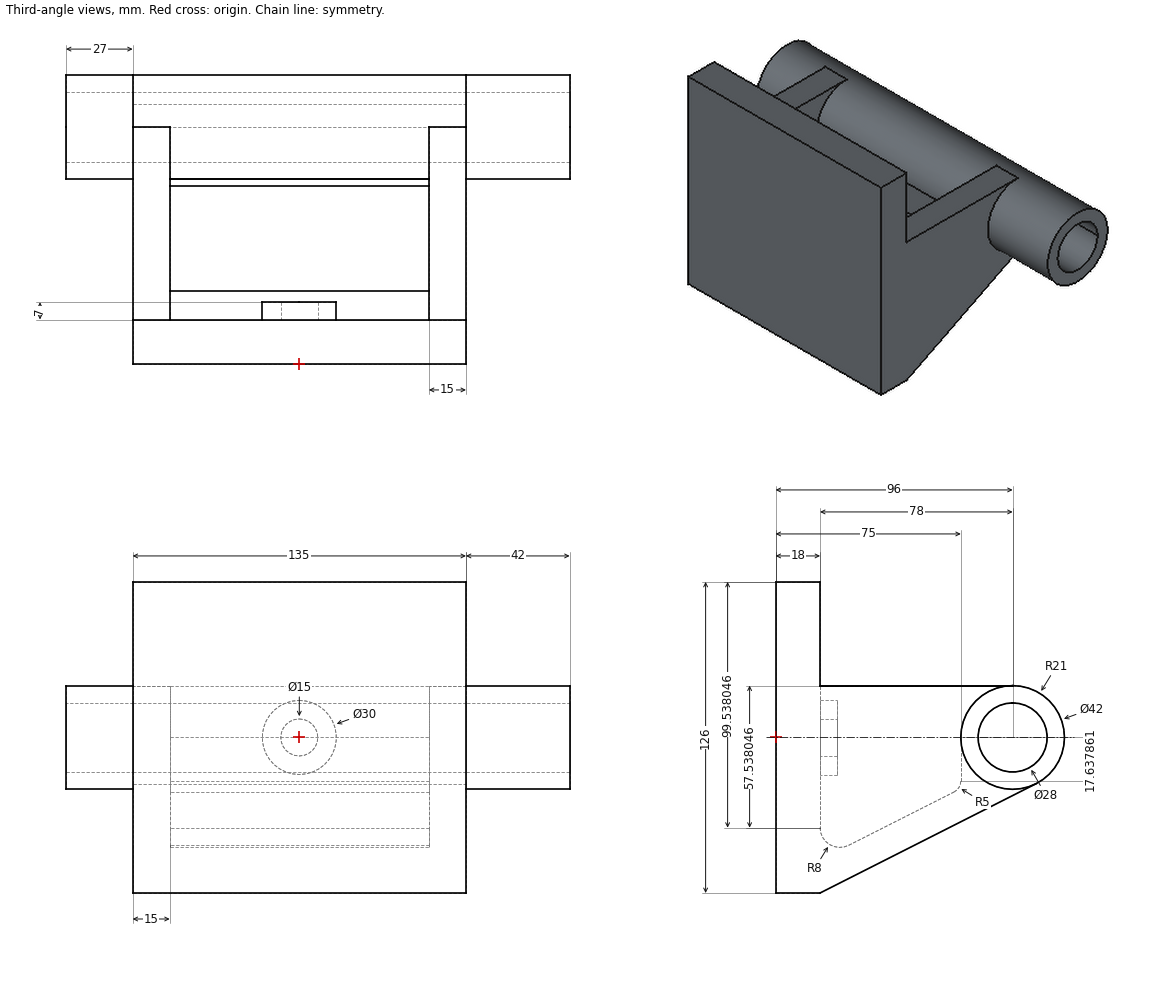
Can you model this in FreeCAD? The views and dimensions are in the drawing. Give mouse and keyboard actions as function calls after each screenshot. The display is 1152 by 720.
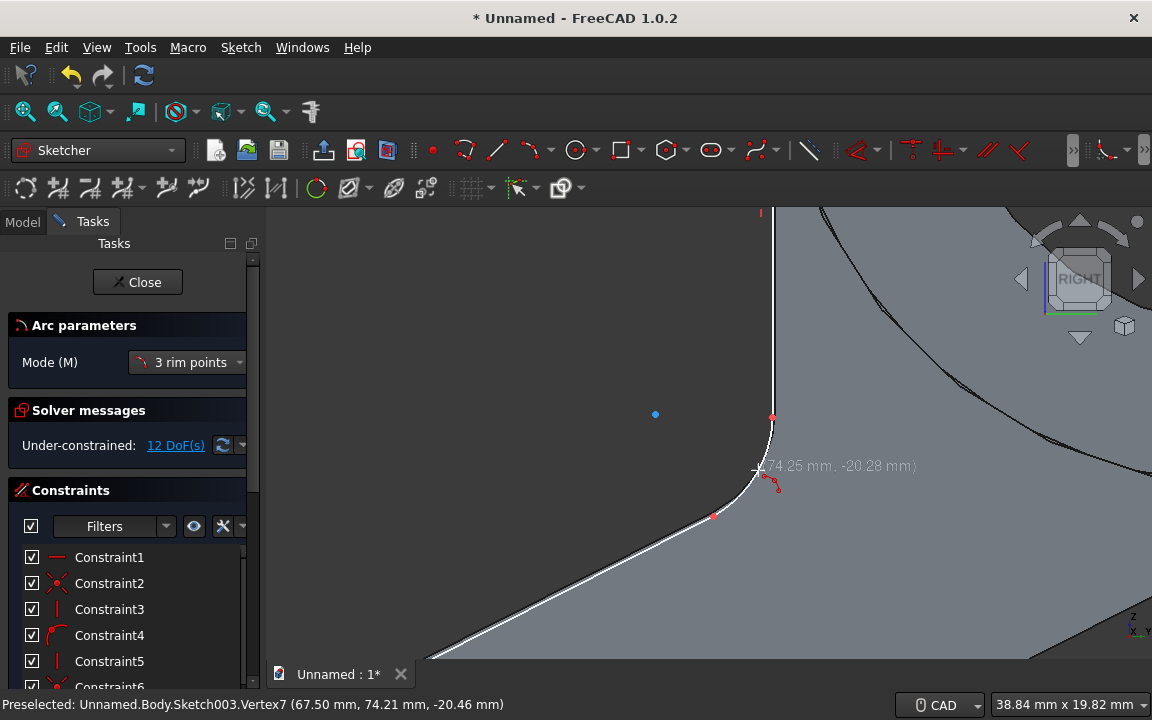
scroll(762, 475, down, 8)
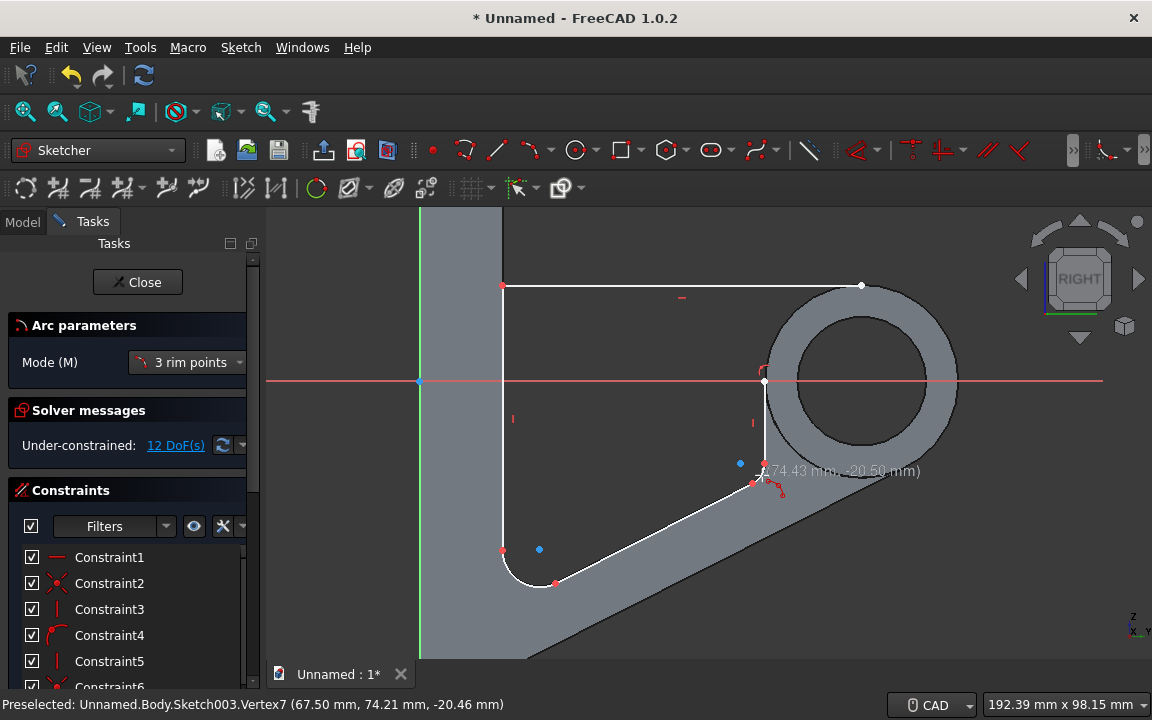
click(765, 381)
click(862, 286)
click(793, 313)
key(Escape)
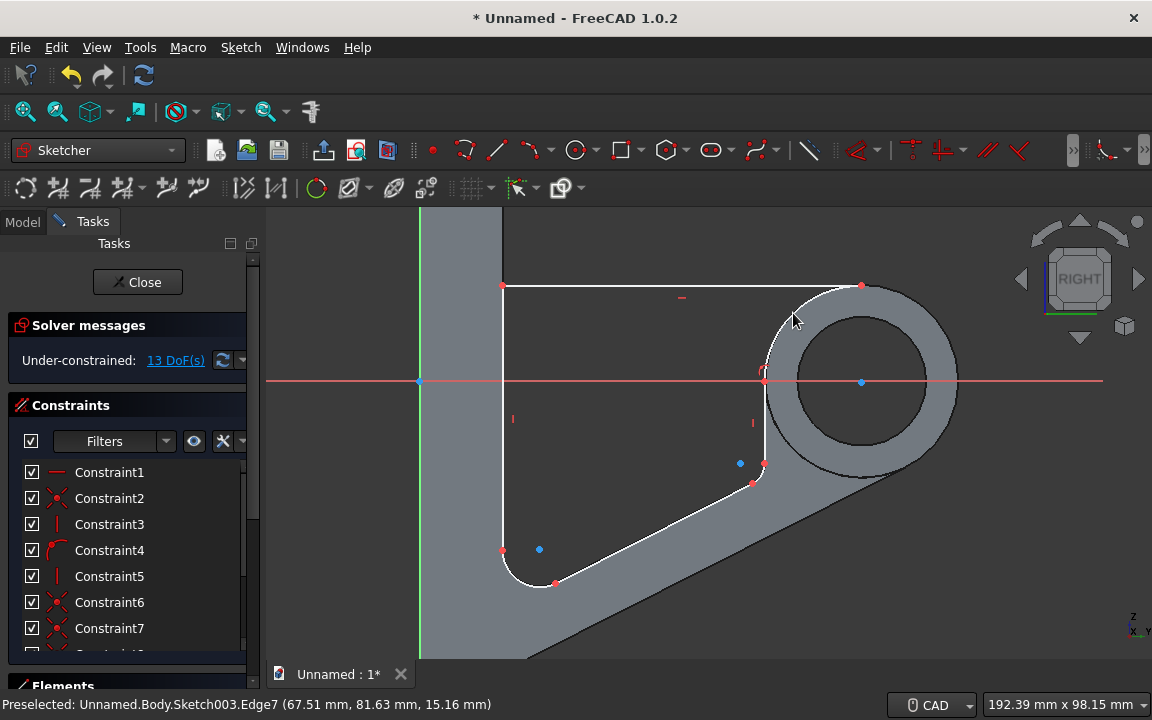
click(754, 286)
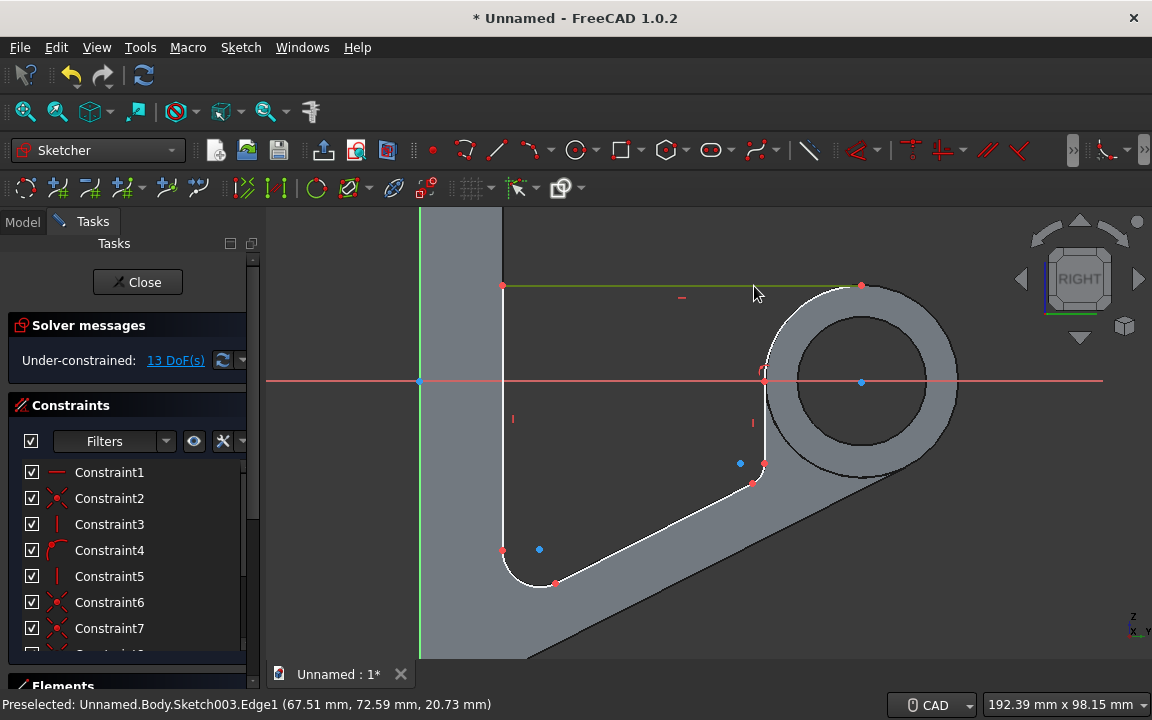
scroll(818, 296, up, 2)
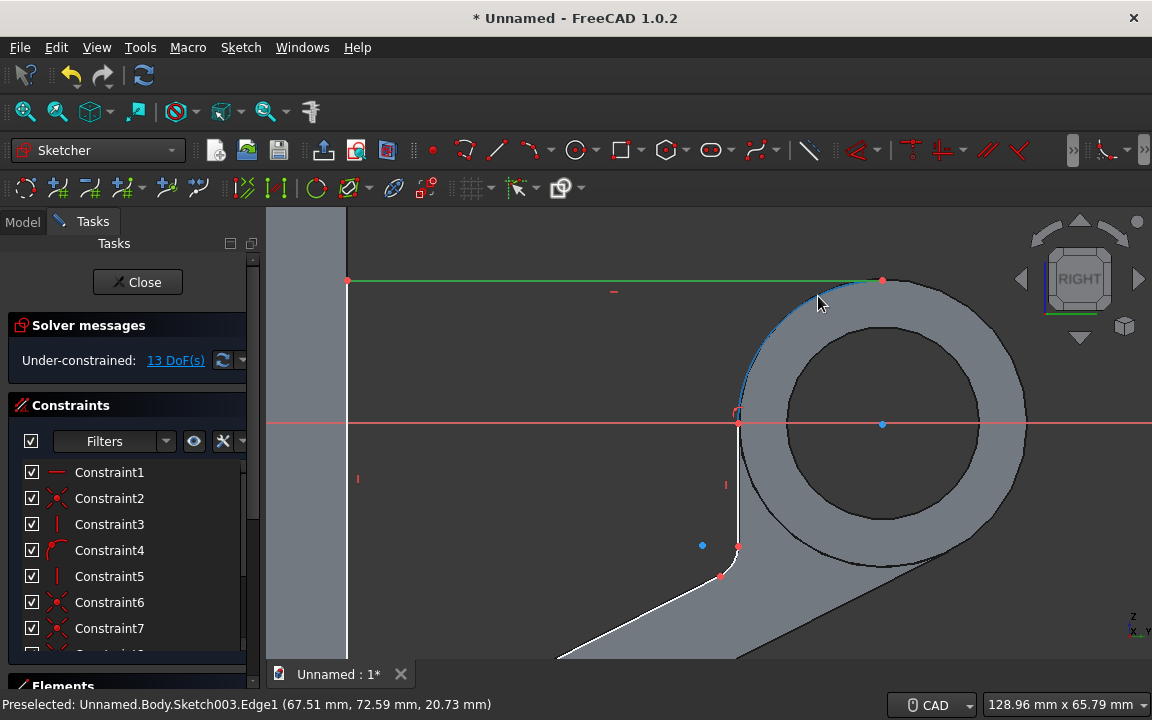
click(818, 296)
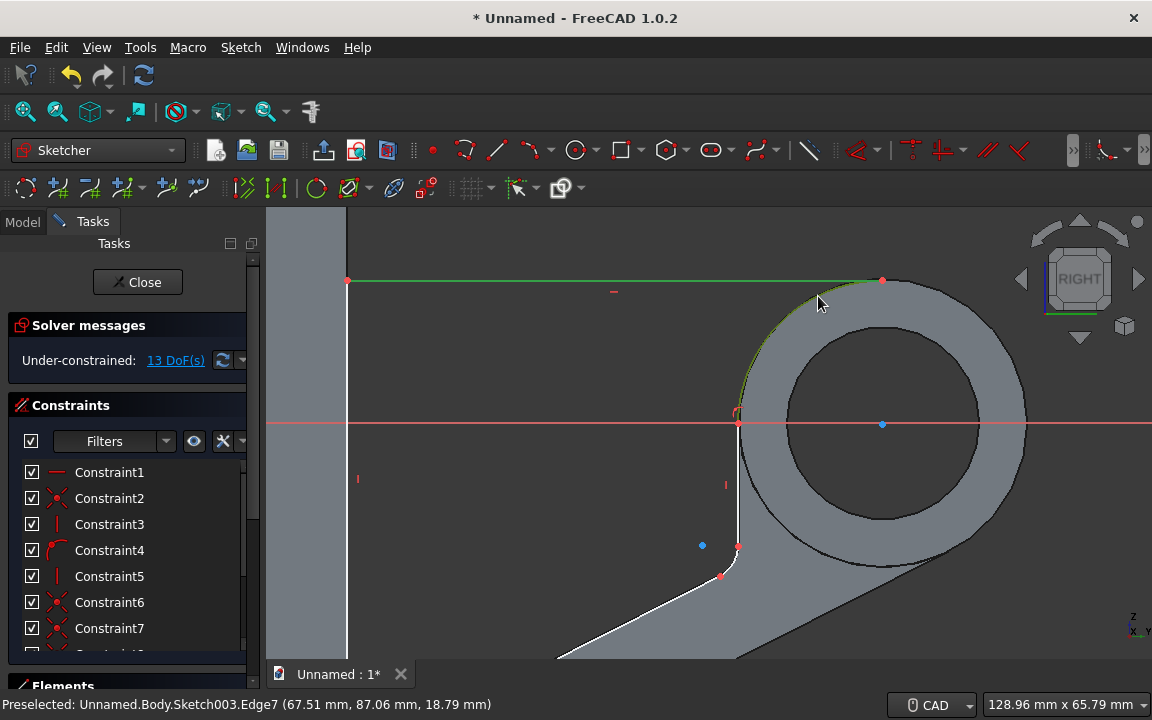
key(t)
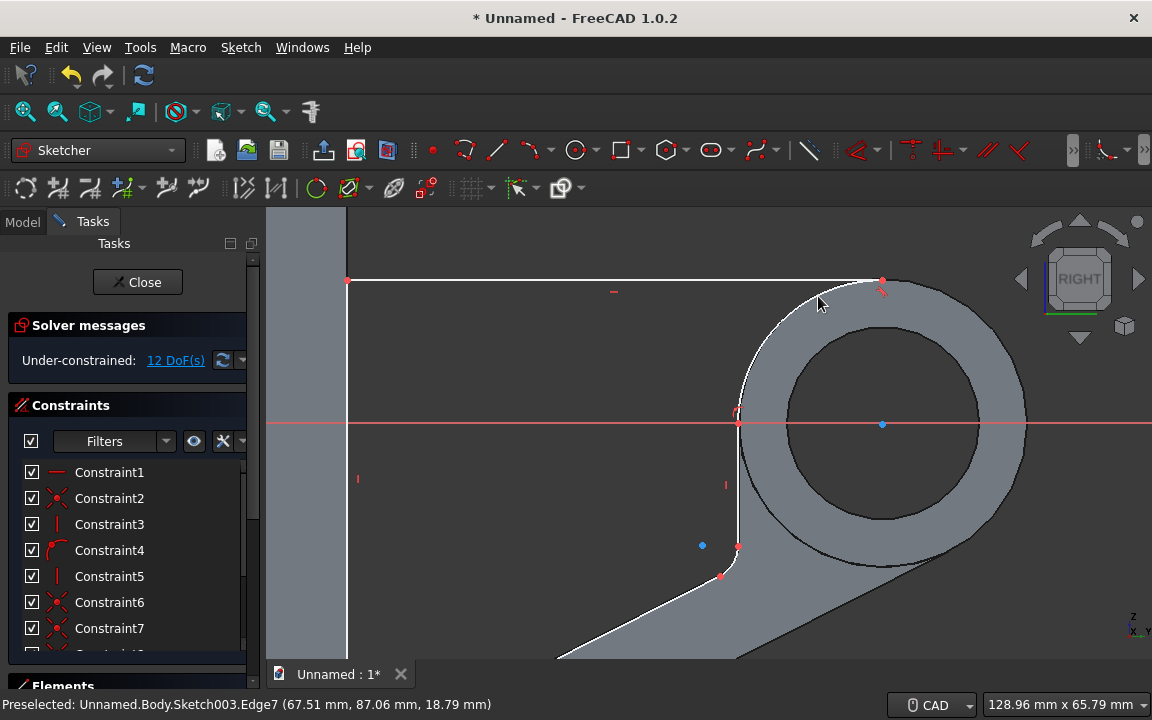
click(347, 399)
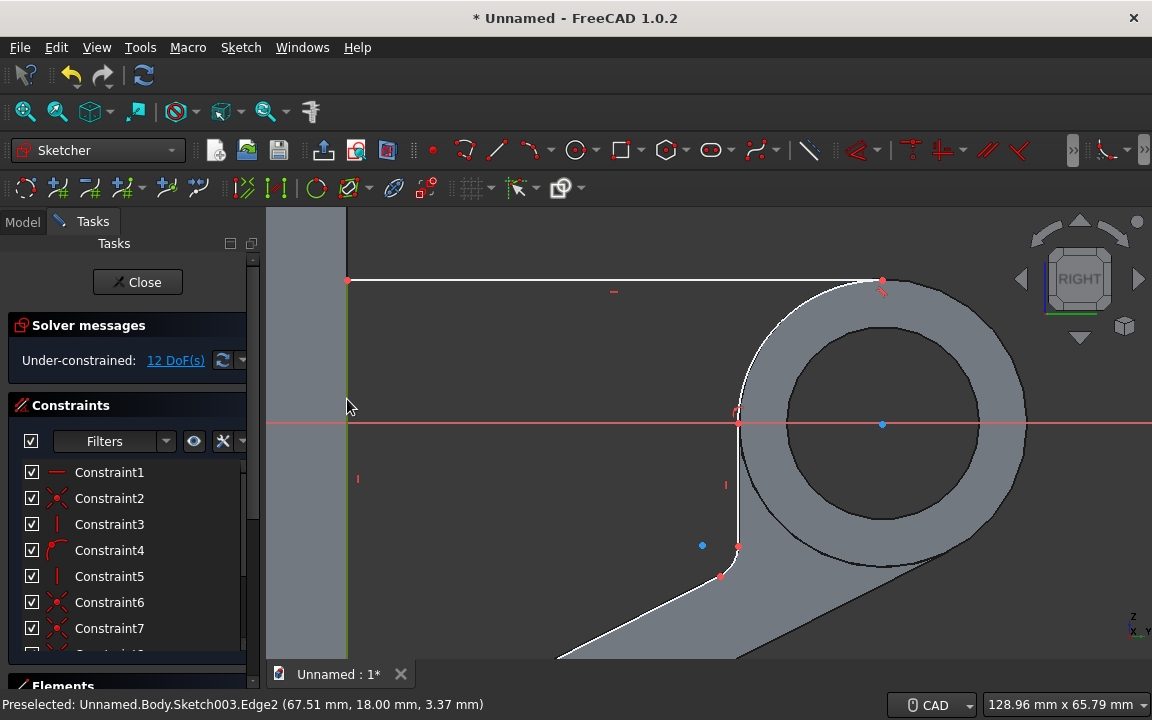
scroll(818, 295, down, 2)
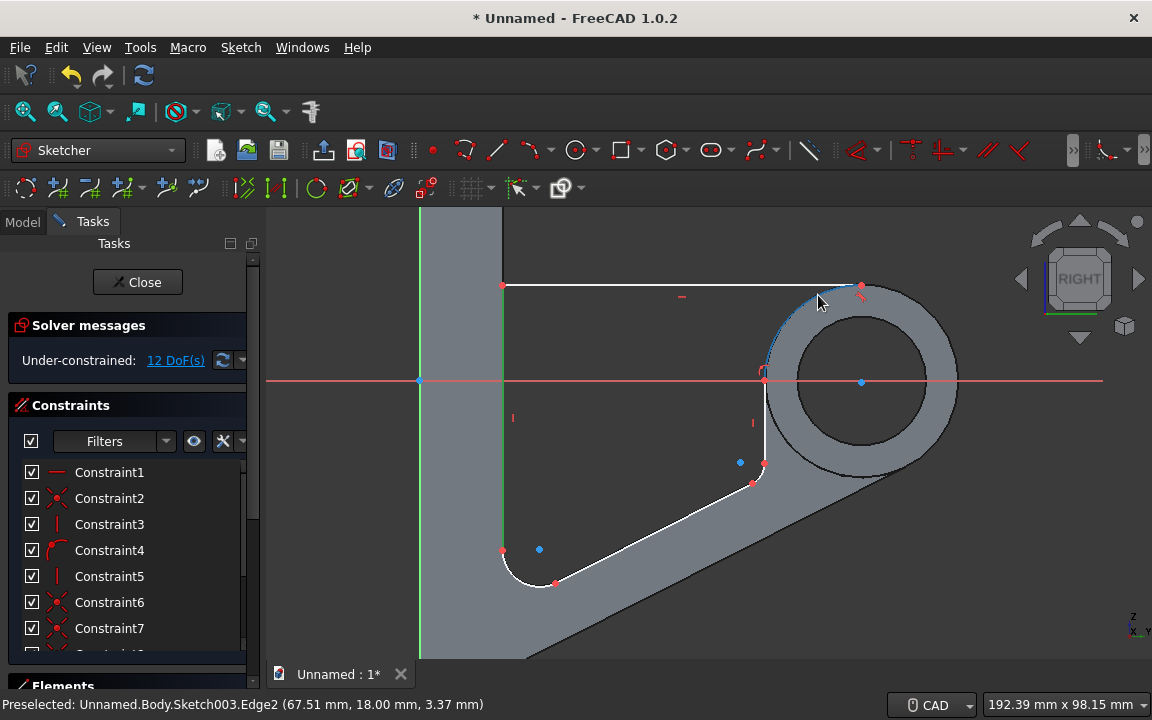
click(510, 571)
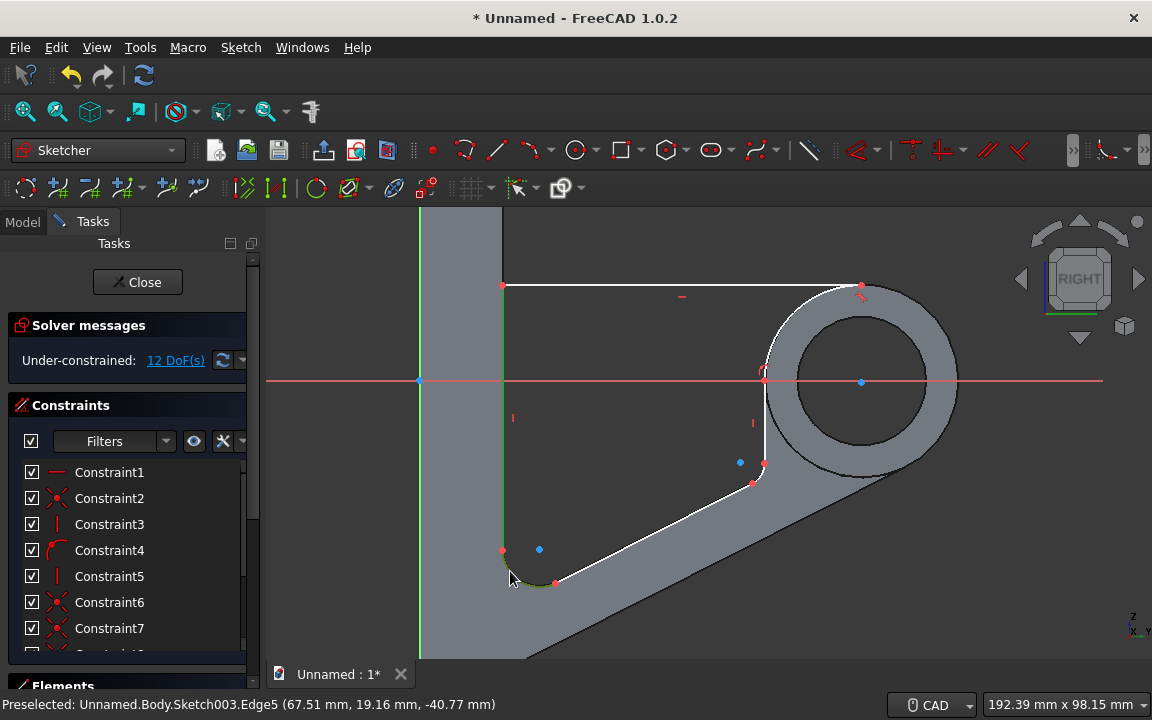
key(t)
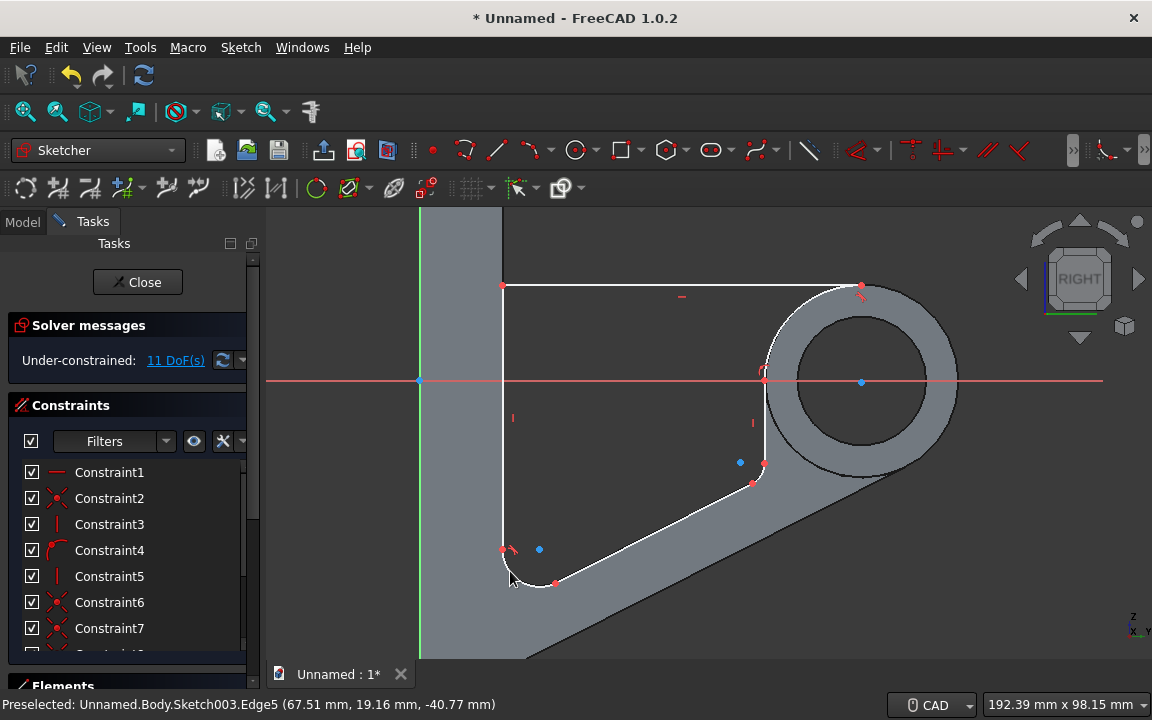
click(615, 553)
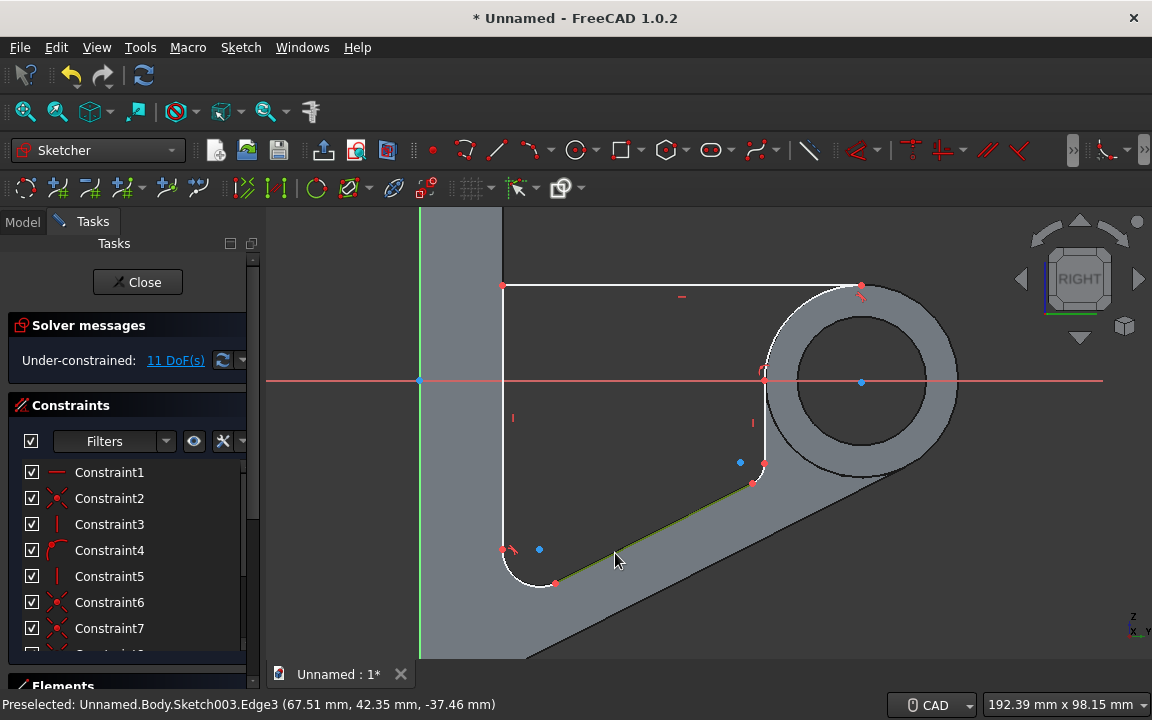
click(509, 571)